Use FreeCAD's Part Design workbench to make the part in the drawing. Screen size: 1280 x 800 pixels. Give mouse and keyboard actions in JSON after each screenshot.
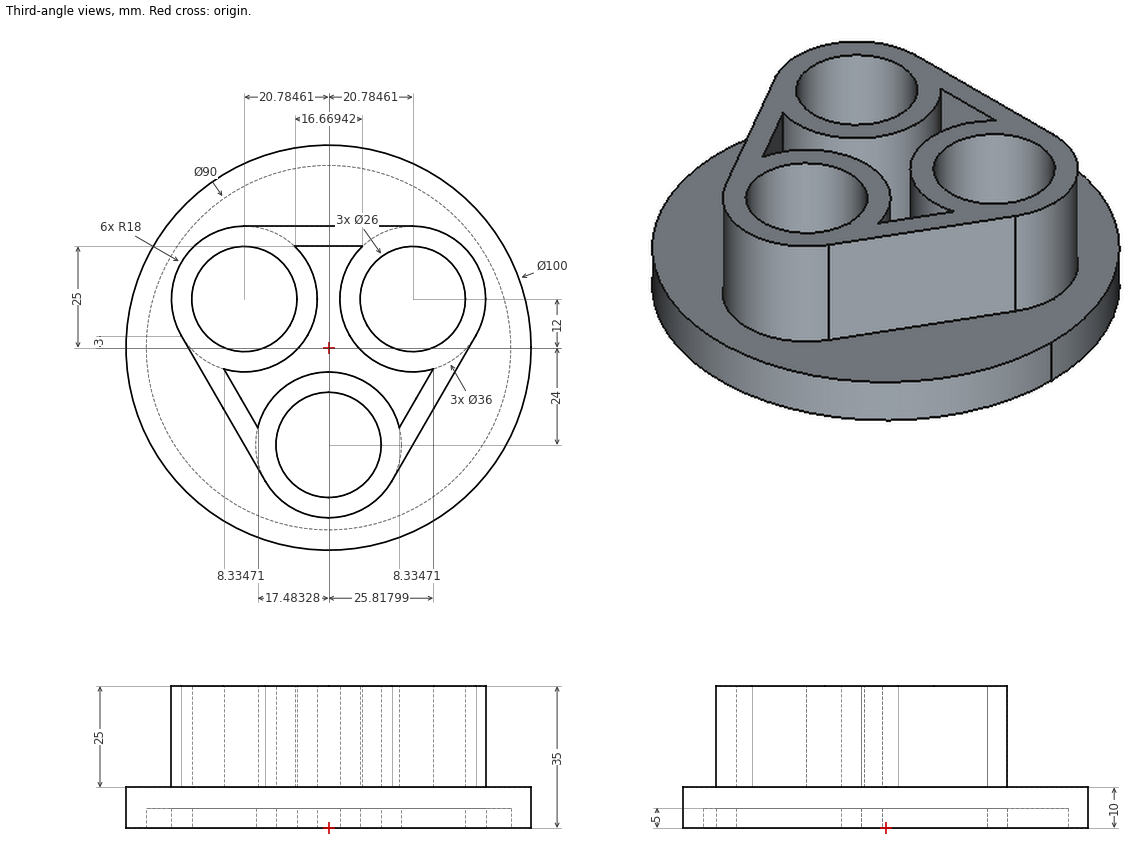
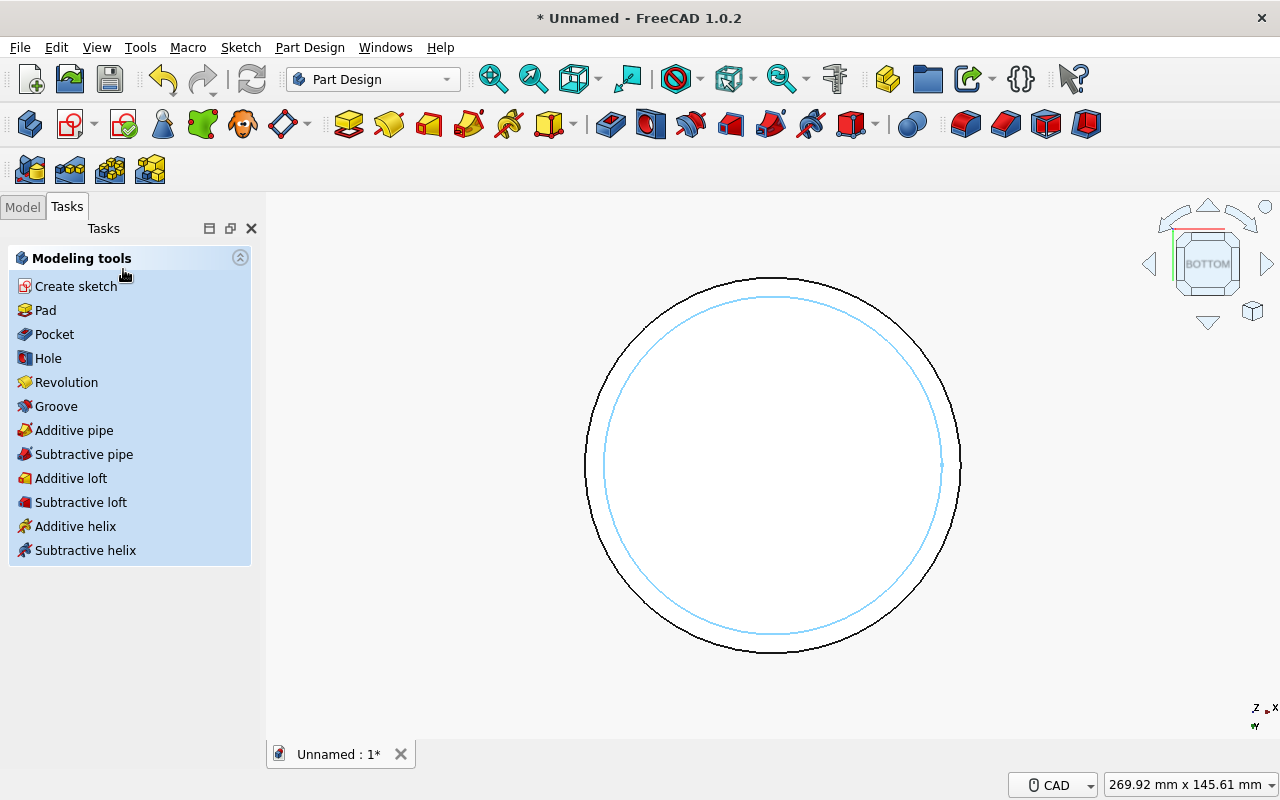
{"action": "left_click", "coordinate": [612, 124]}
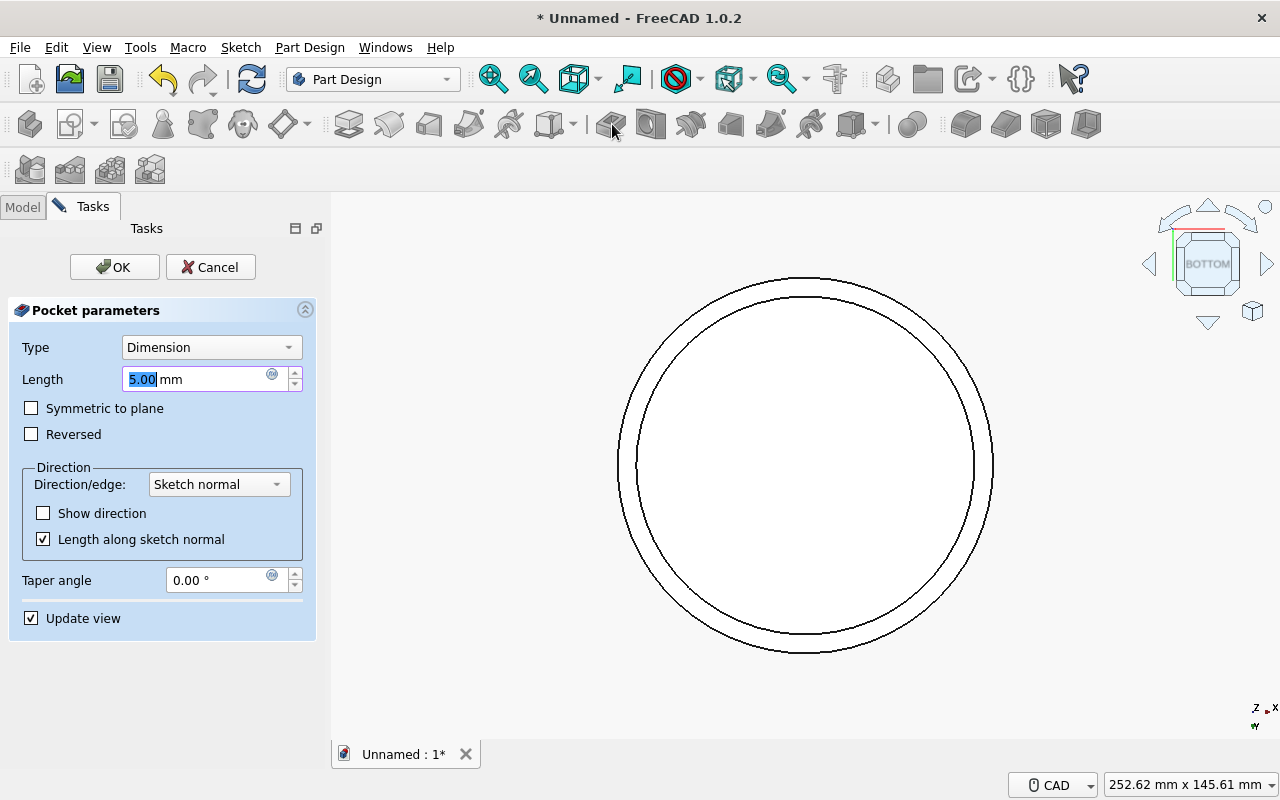
{"action": "type", "text": "5"}
{"action": "key", "text": "Tab"}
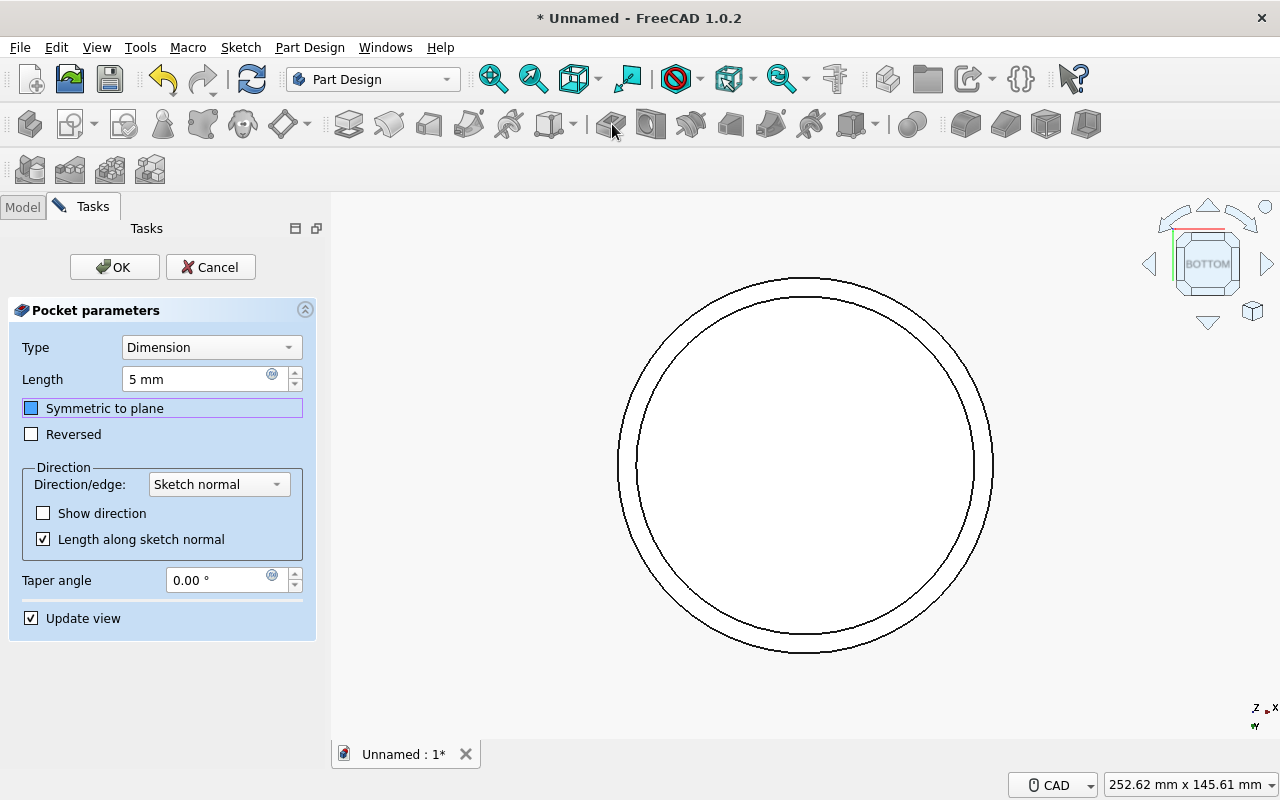
{"action": "left_click", "coordinate": [115, 267]}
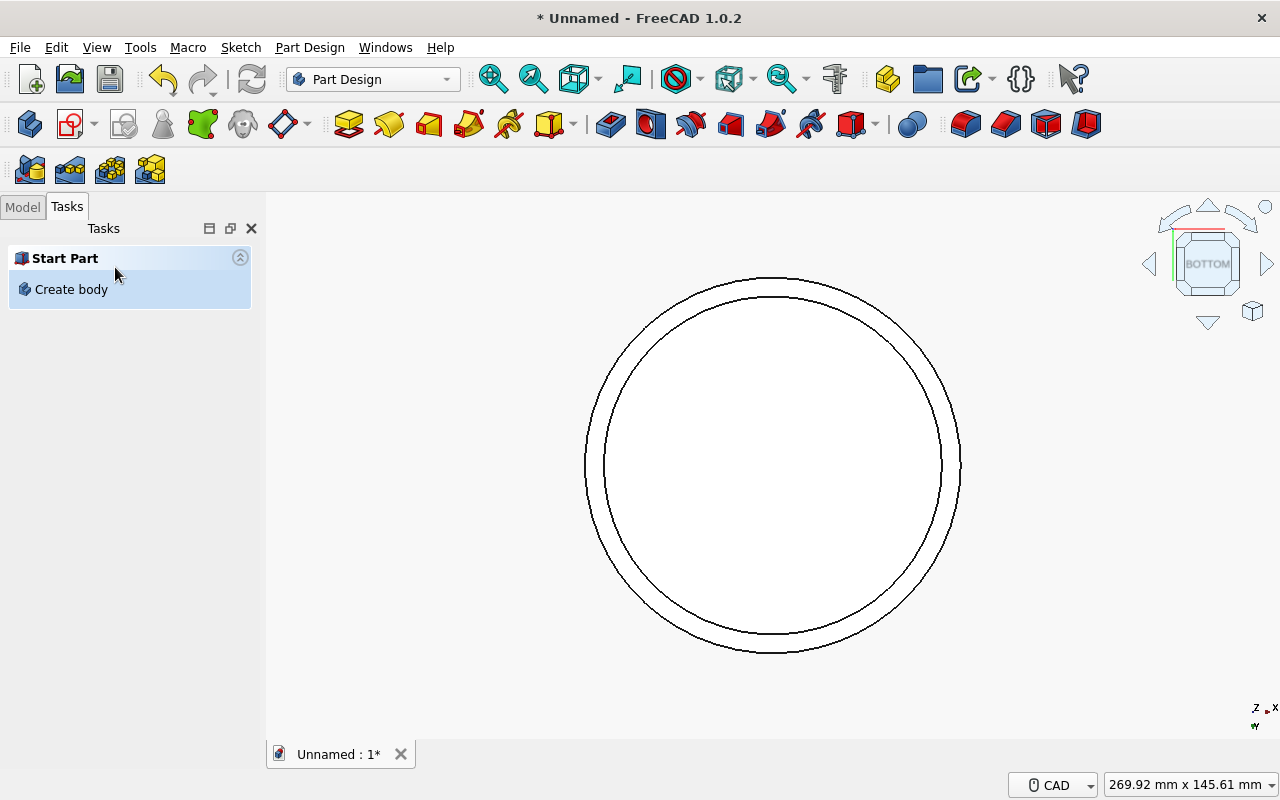
{"action": "scroll", "coordinate": [934, 518], "scroll_direction": "up", "scroll_amount": 15}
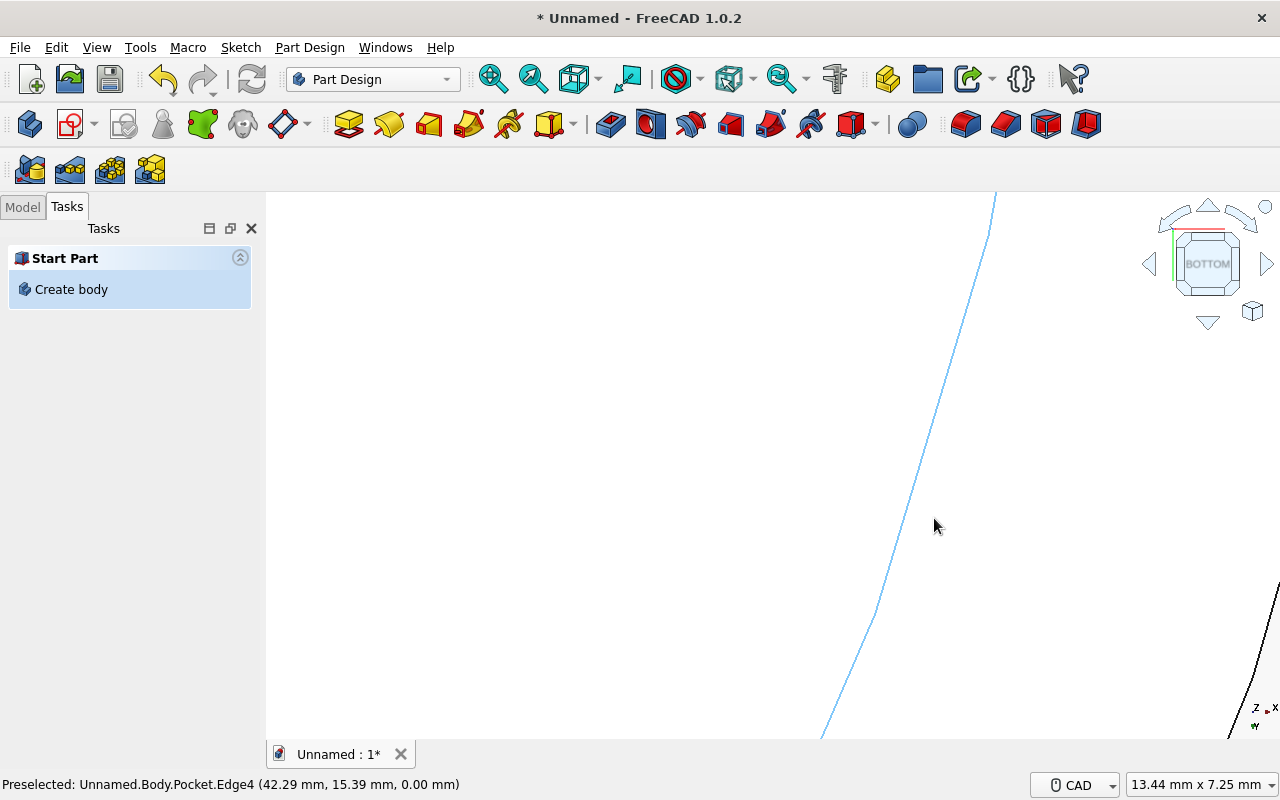
{"action": "left_click", "coordinate": [919, 529]}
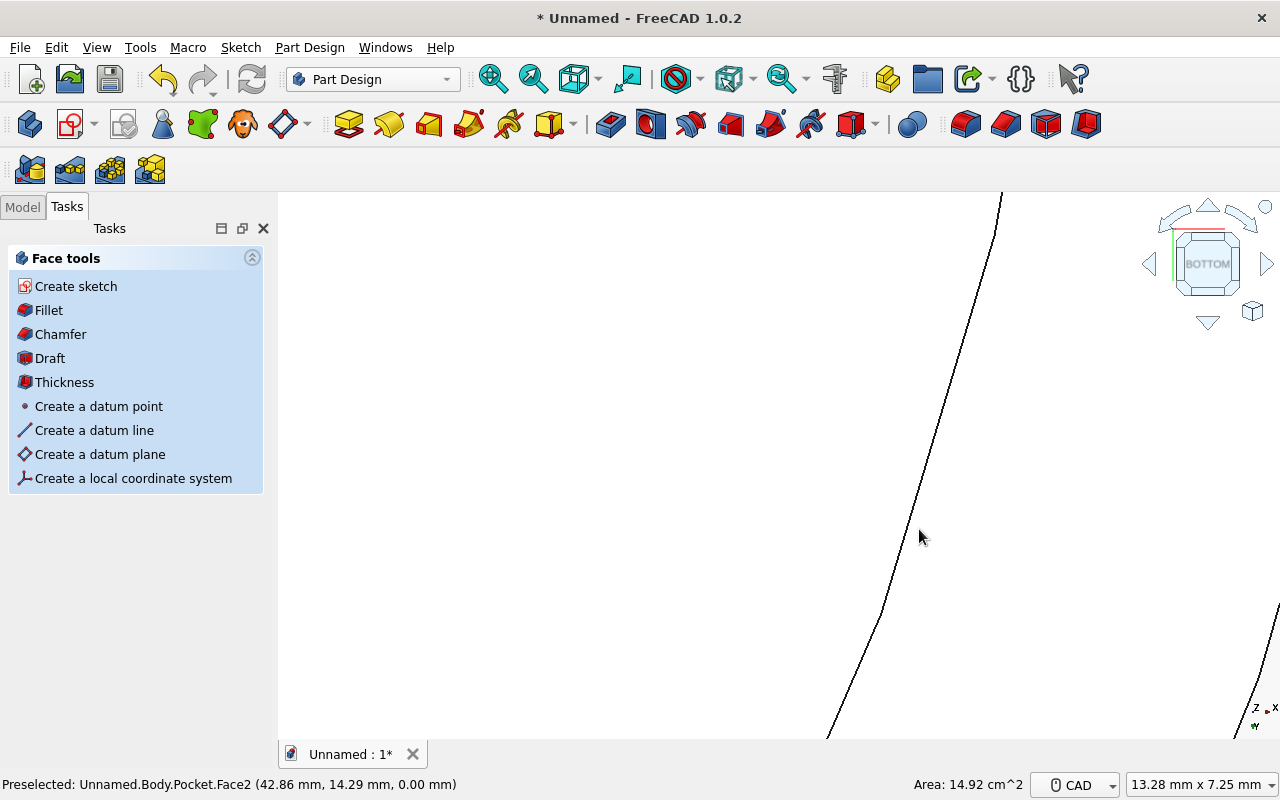
{"action": "left_click", "coordinate": [70, 124]}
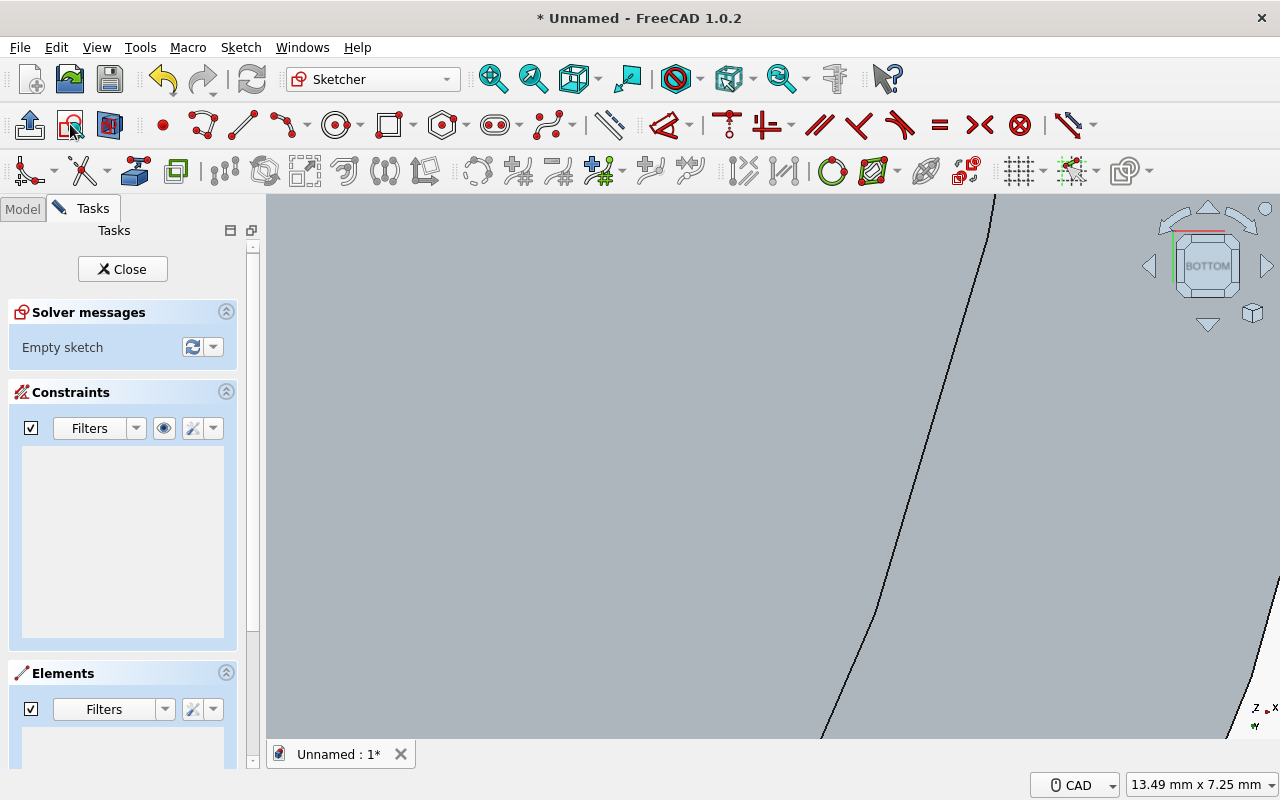
{"action": "scroll", "coordinate": [899, 561], "scroll_direction": "down", "scroll_amount": 14}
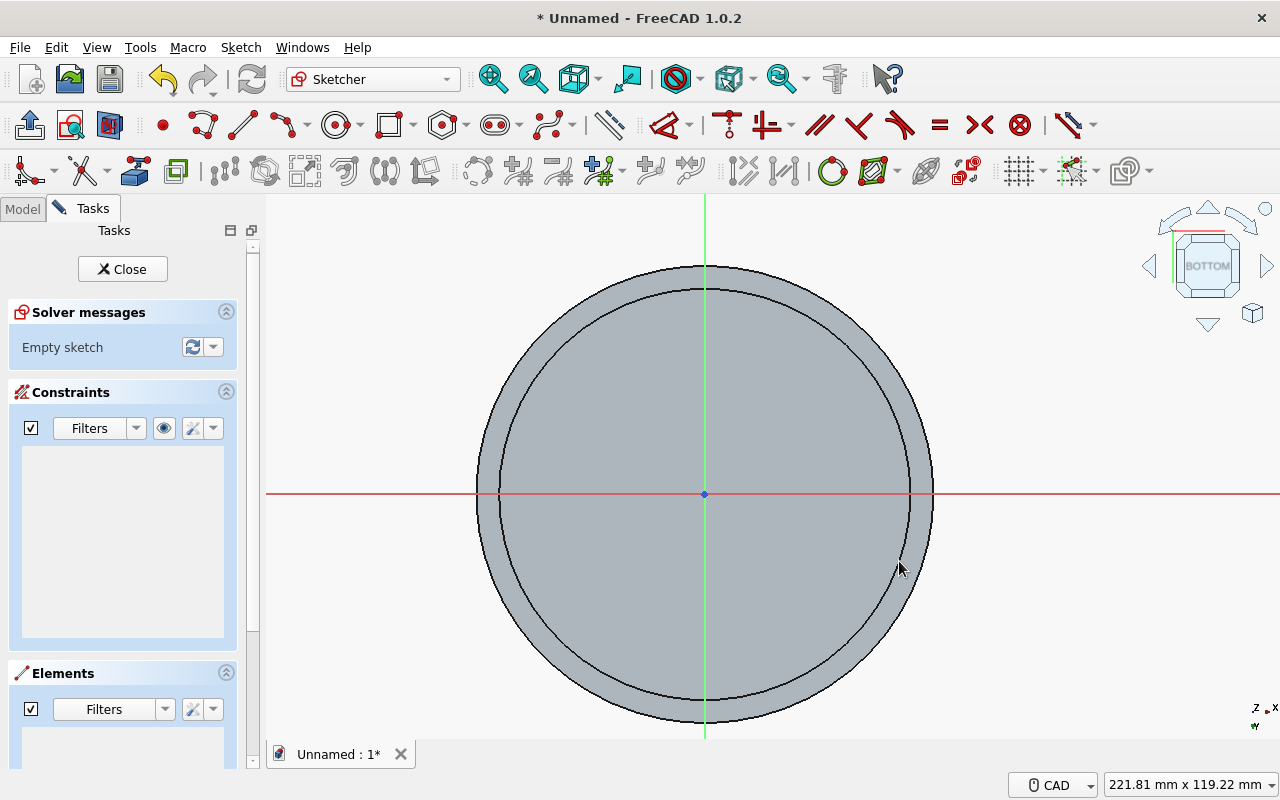
{"action": "left_click", "coordinate": [336, 126]}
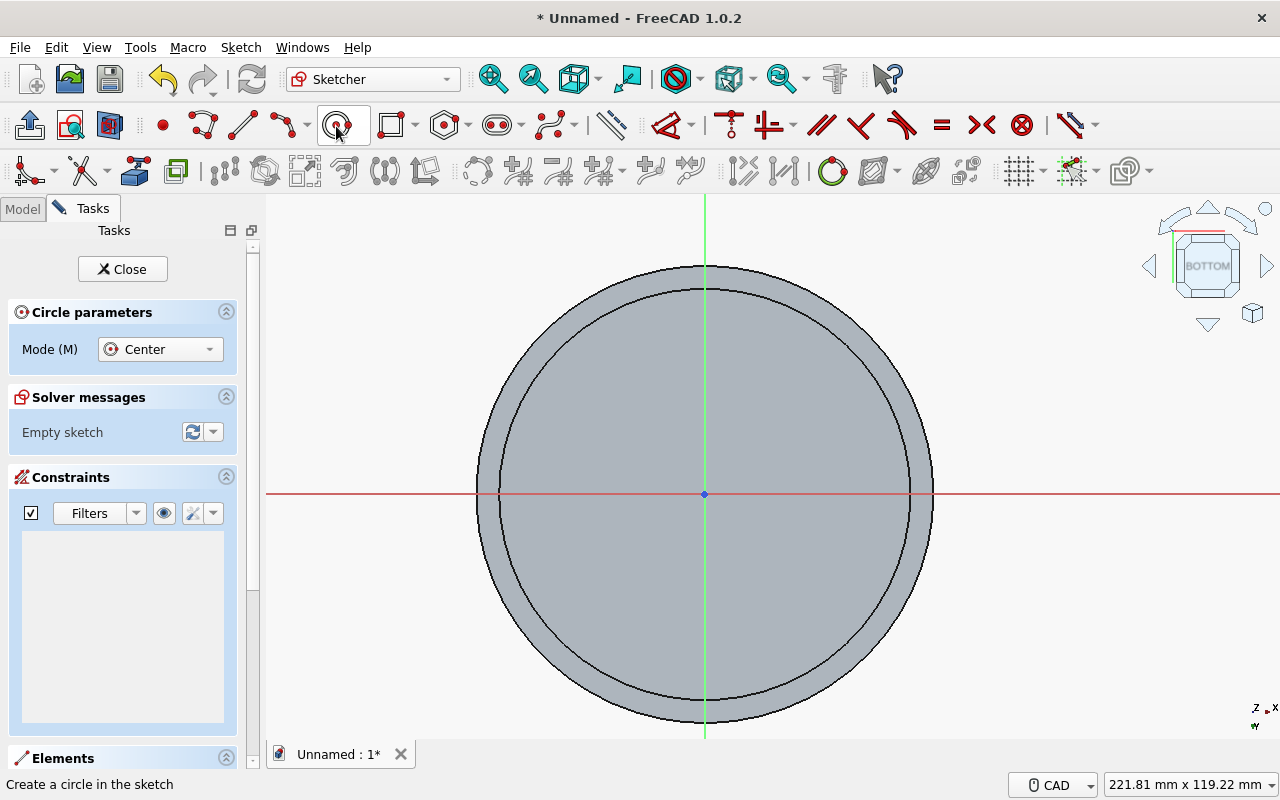
{"action": "left_click", "coordinate": [800, 549]}
{"action": "left_click", "coordinate": [858, 608]}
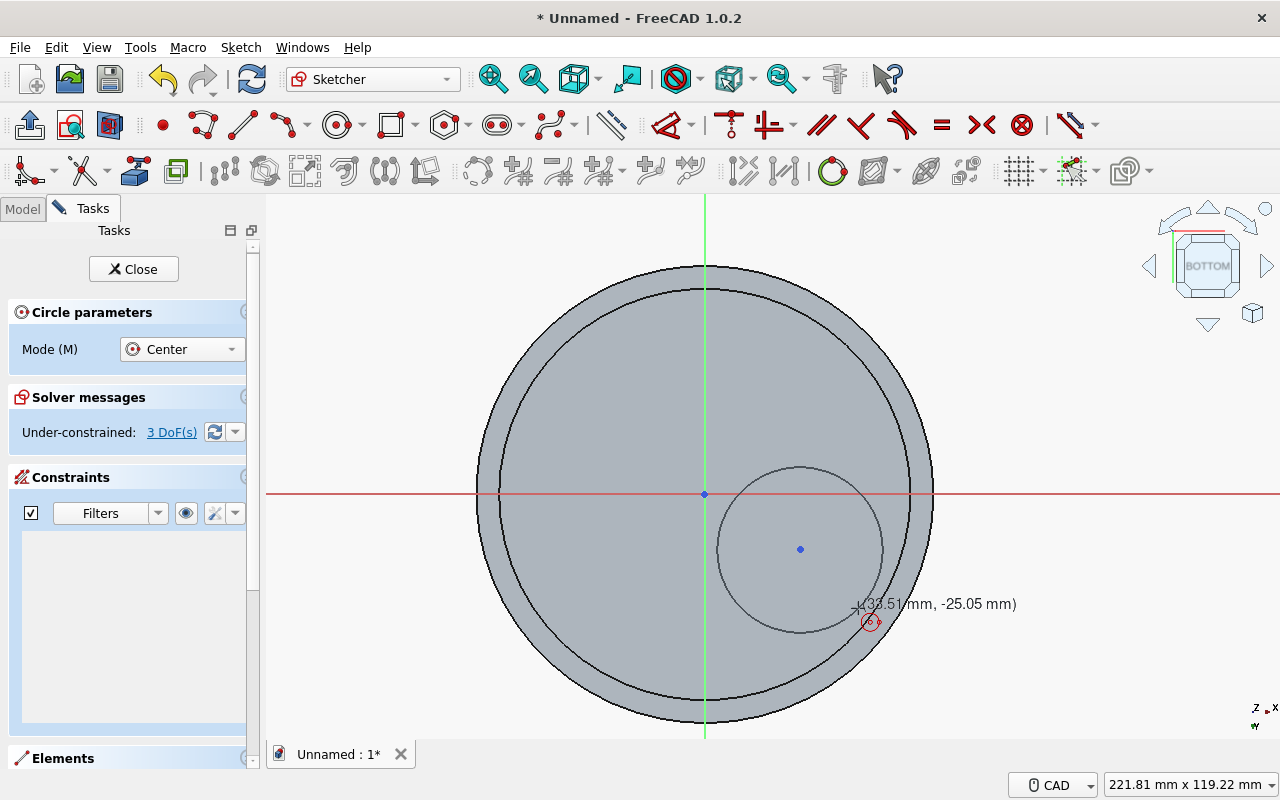
{"action": "left_click", "coordinate": [610, 549]}
{"action": "left_click", "coordinate": [668, 608]}